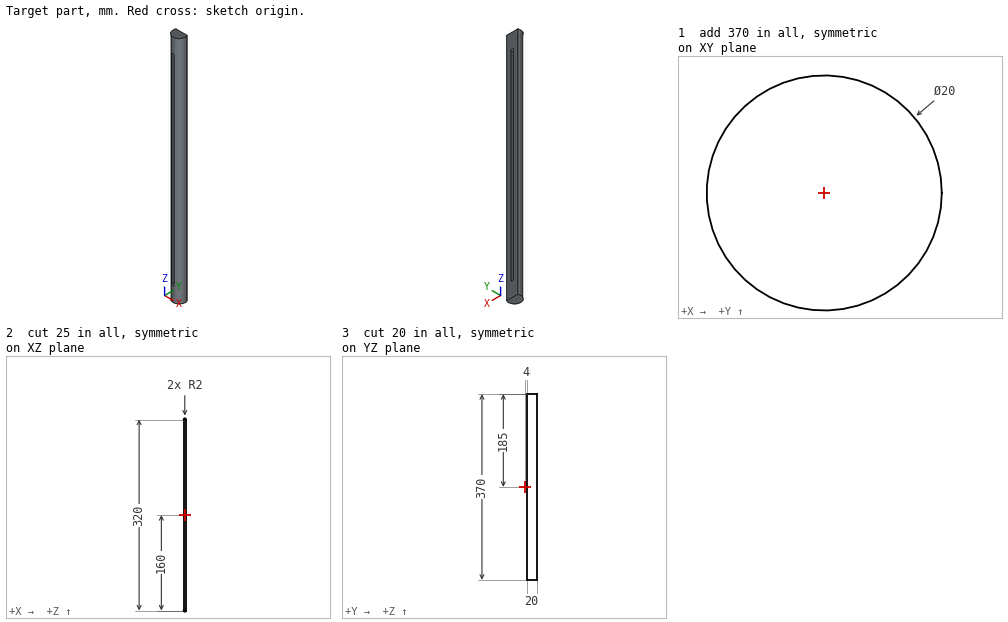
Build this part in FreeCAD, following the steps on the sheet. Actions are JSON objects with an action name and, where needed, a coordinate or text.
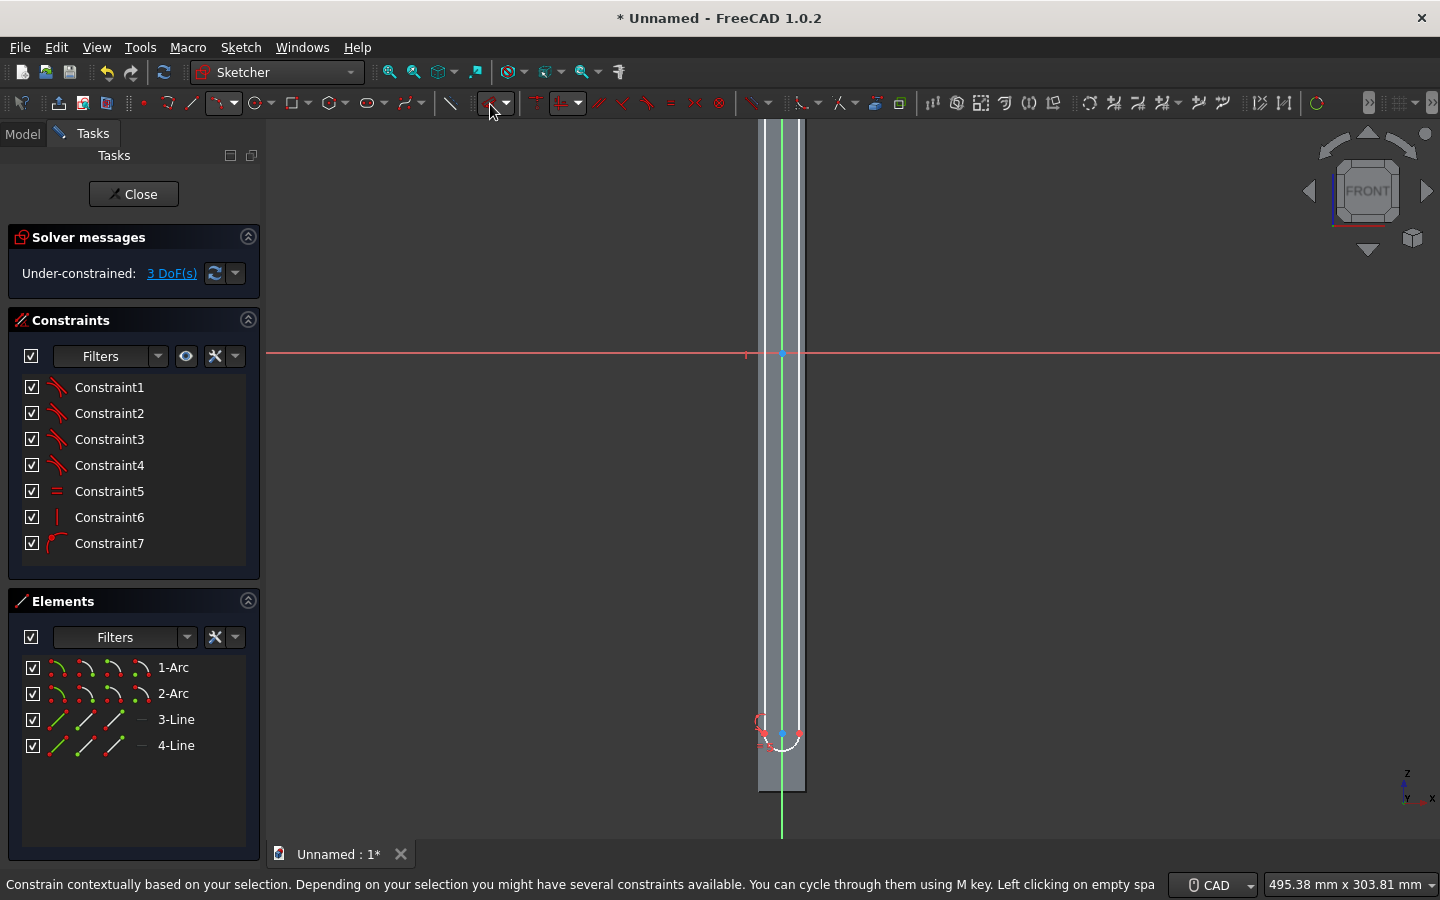
{"action": "scroll", "coordinate": [772, 748], "scroll_direction": "up", "scroll_amount": 11}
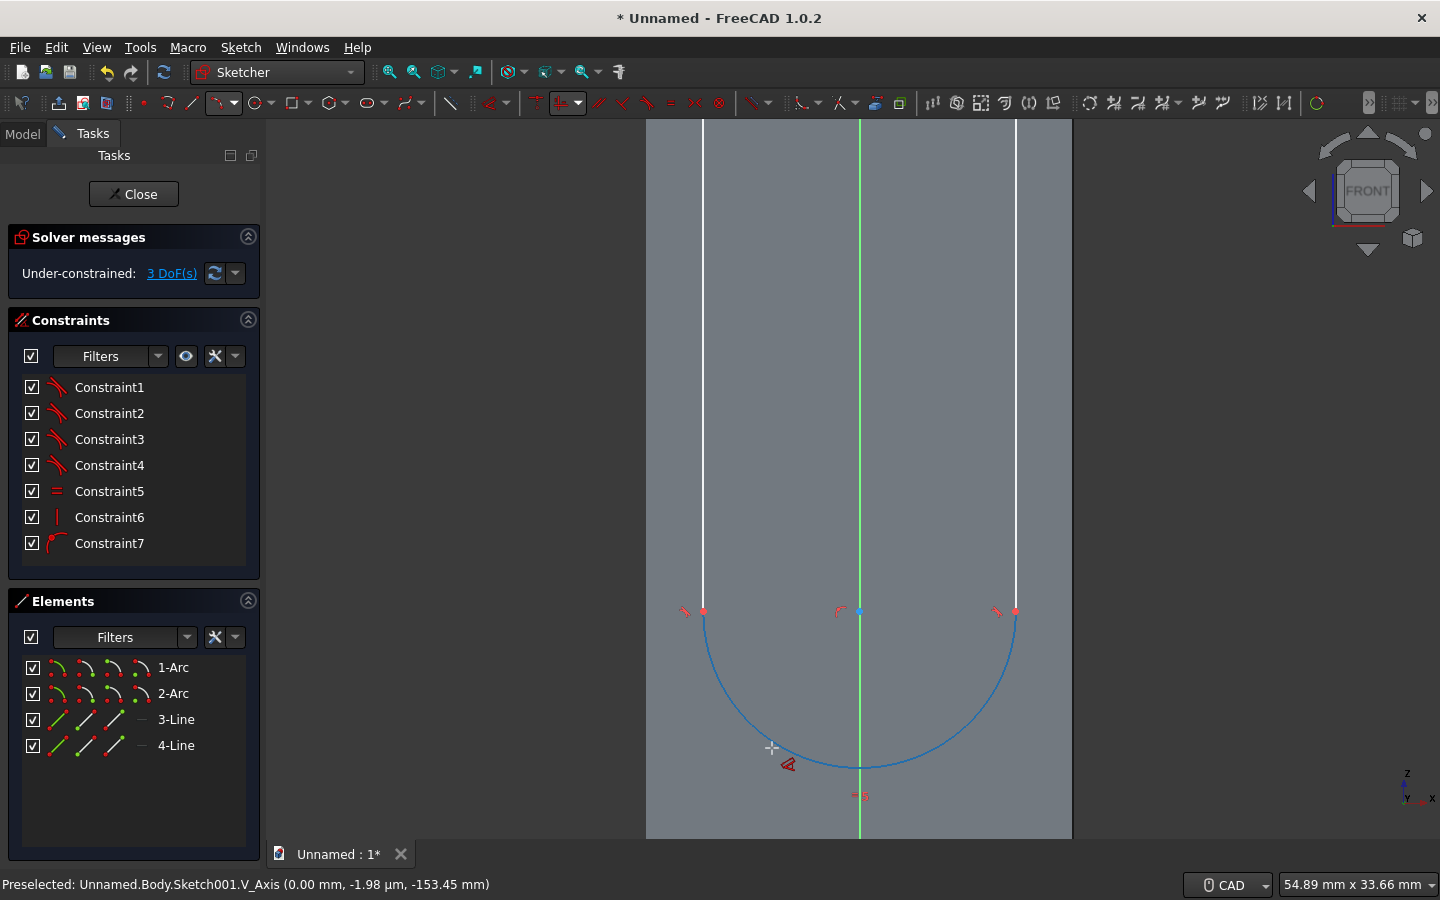
{"action": "left_click", "coordinate": [768, 738]}
{"action": "left_click", "coordinate": [749, 764]}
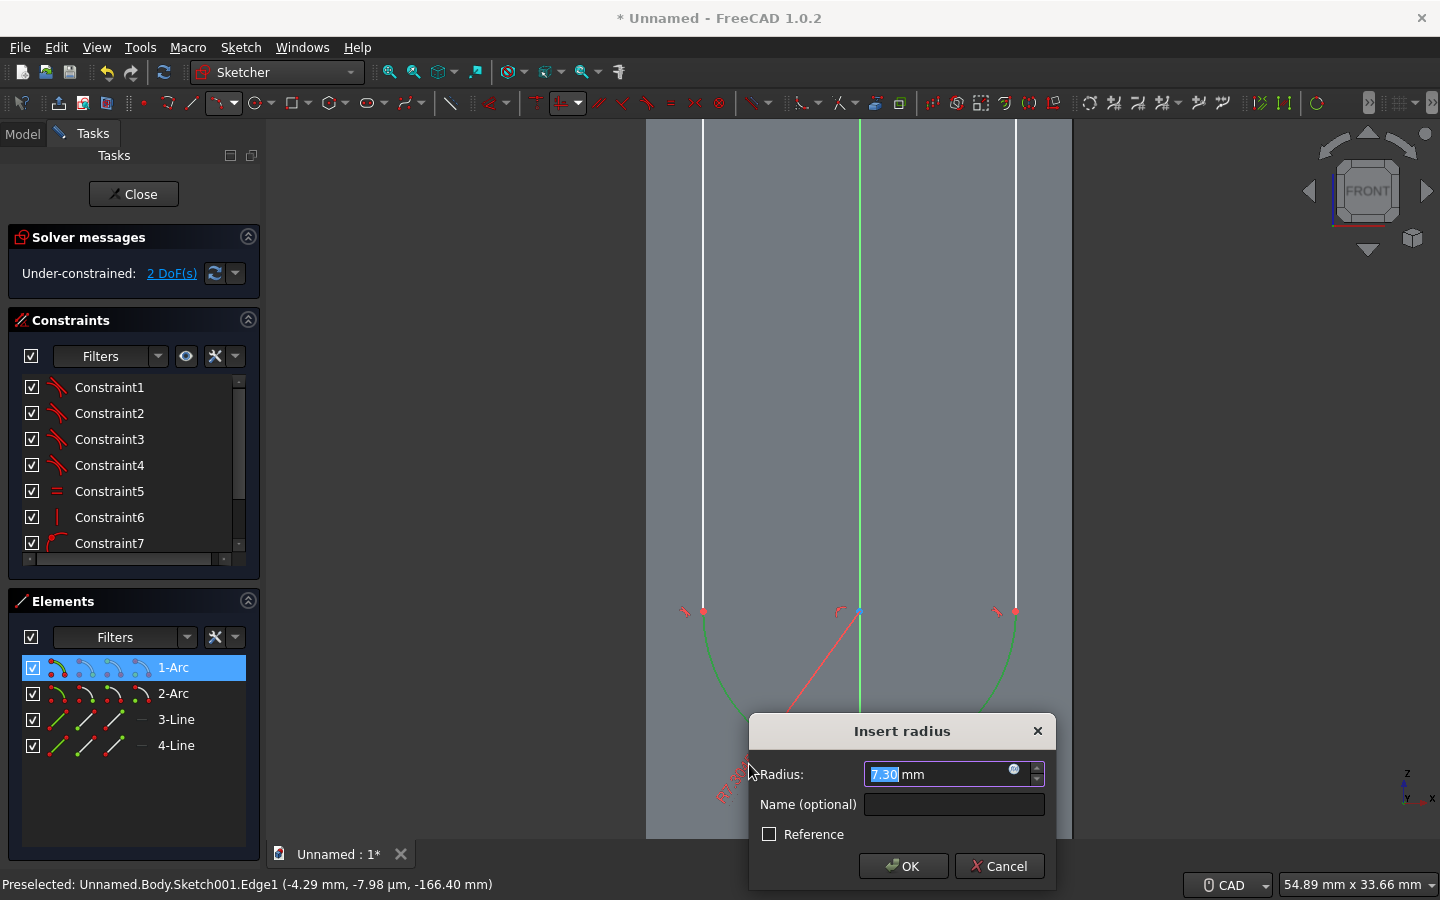
{"action": "type", "text": "2"}
{"action": "key", "text": "Return"}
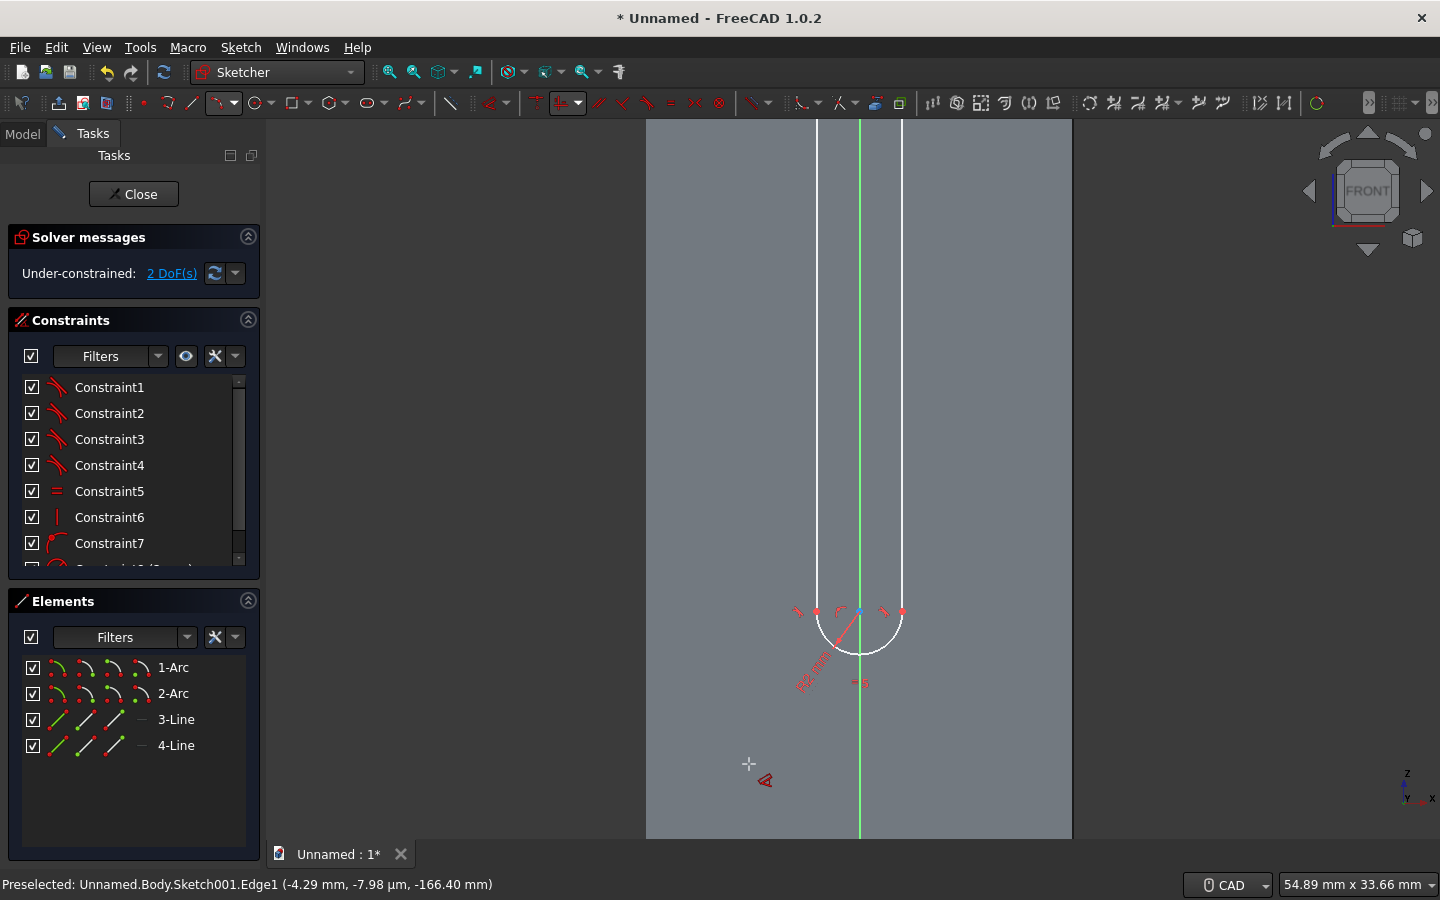
{"action": "scroll", "coordinate": [778, 744], "scroll_direction": "down", "scroll_amount": 13}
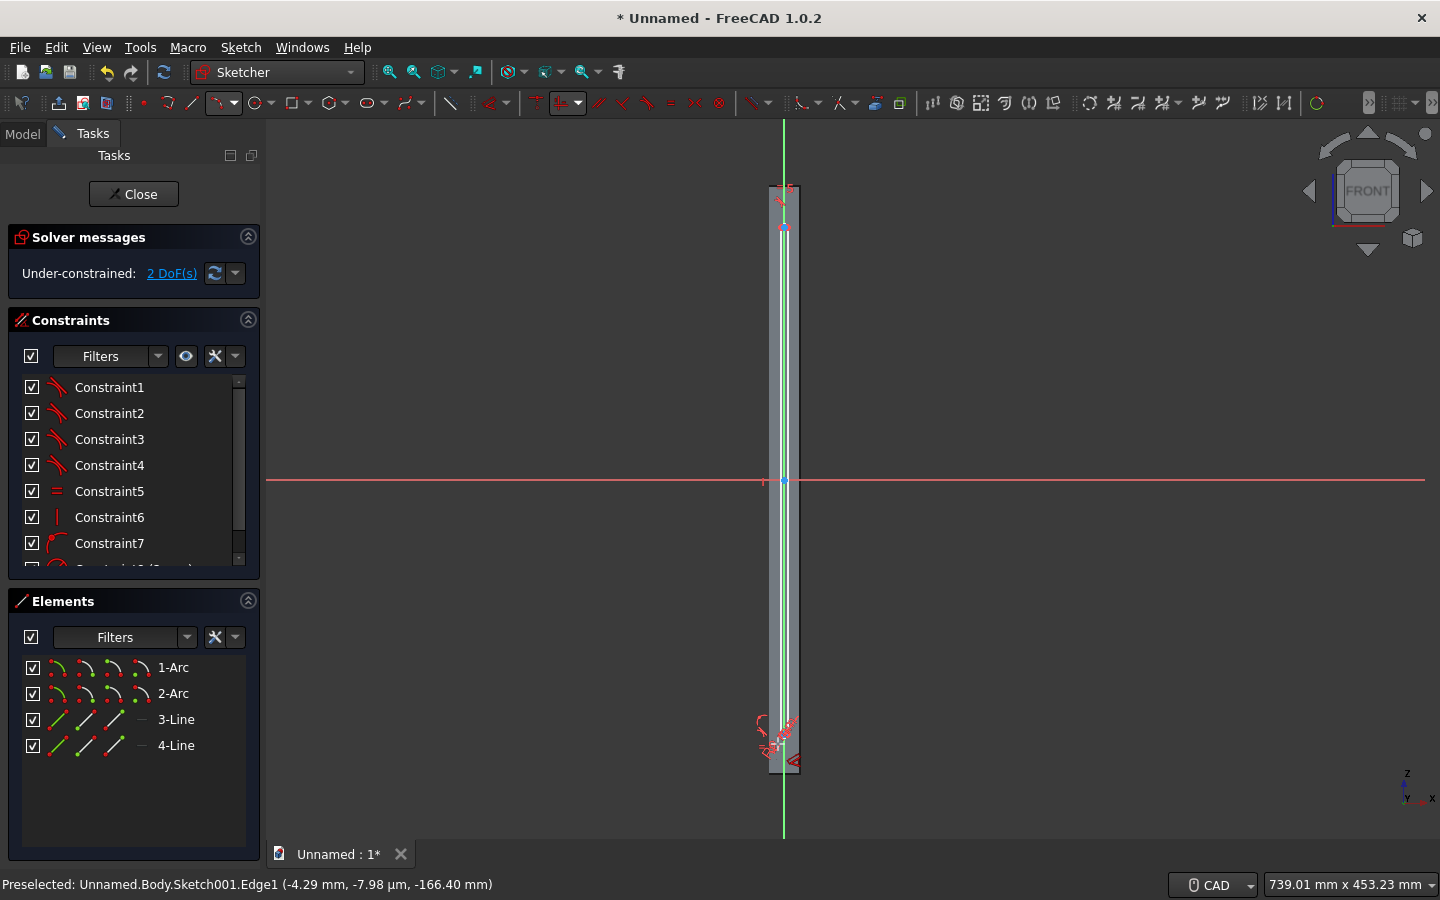
{"action": "scroll", "coordinate": [781, 583], "scroll_direction": "up", "scroll_amount": 8}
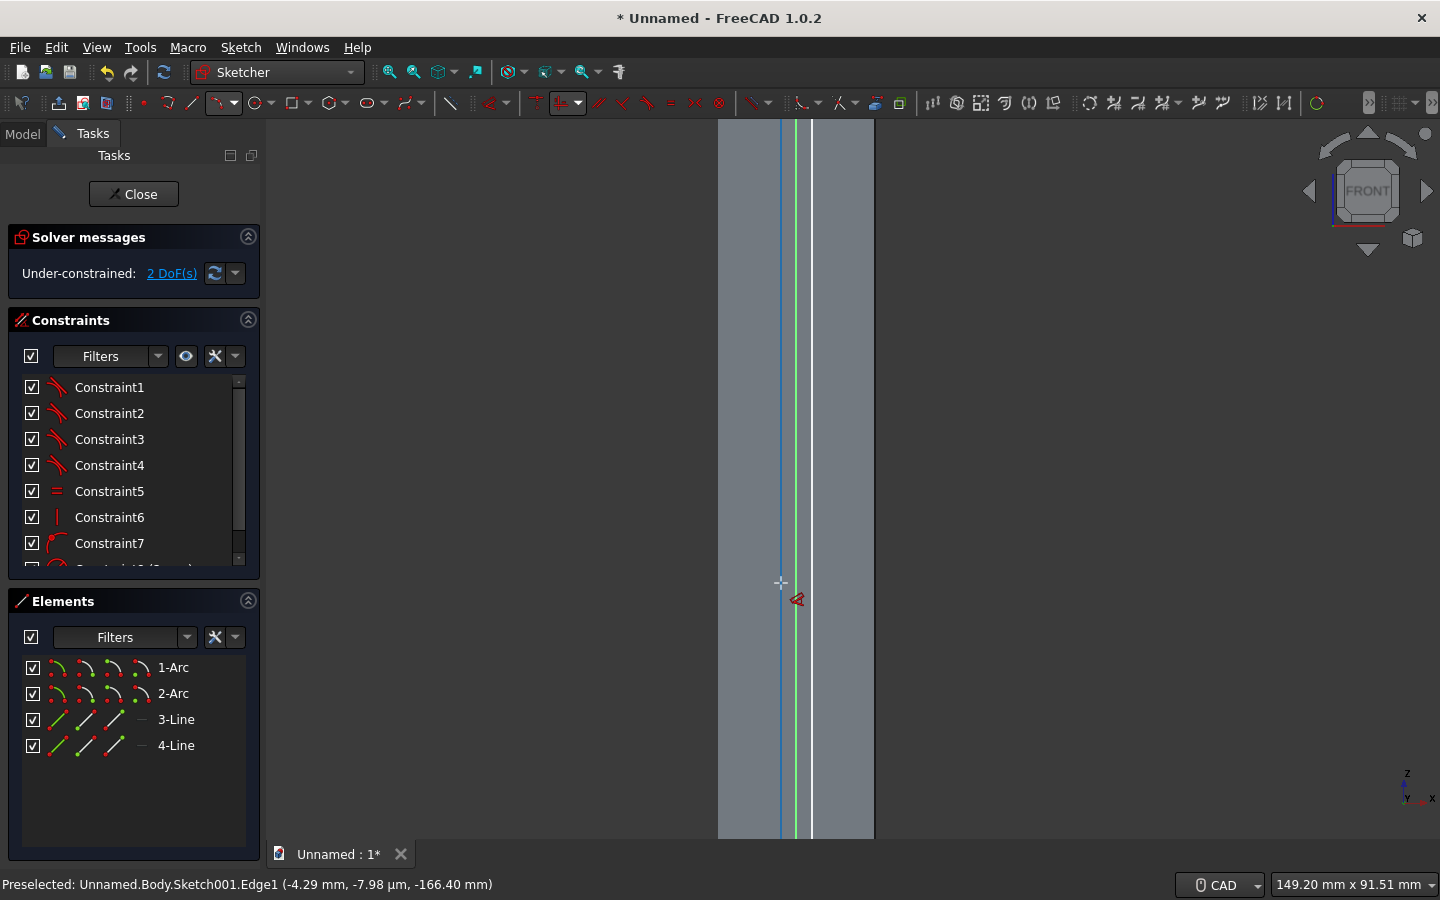
{"action": "left_click", "coordinate": [781, 579]}
{"action": "left_click", "coordinate": [747, 479]}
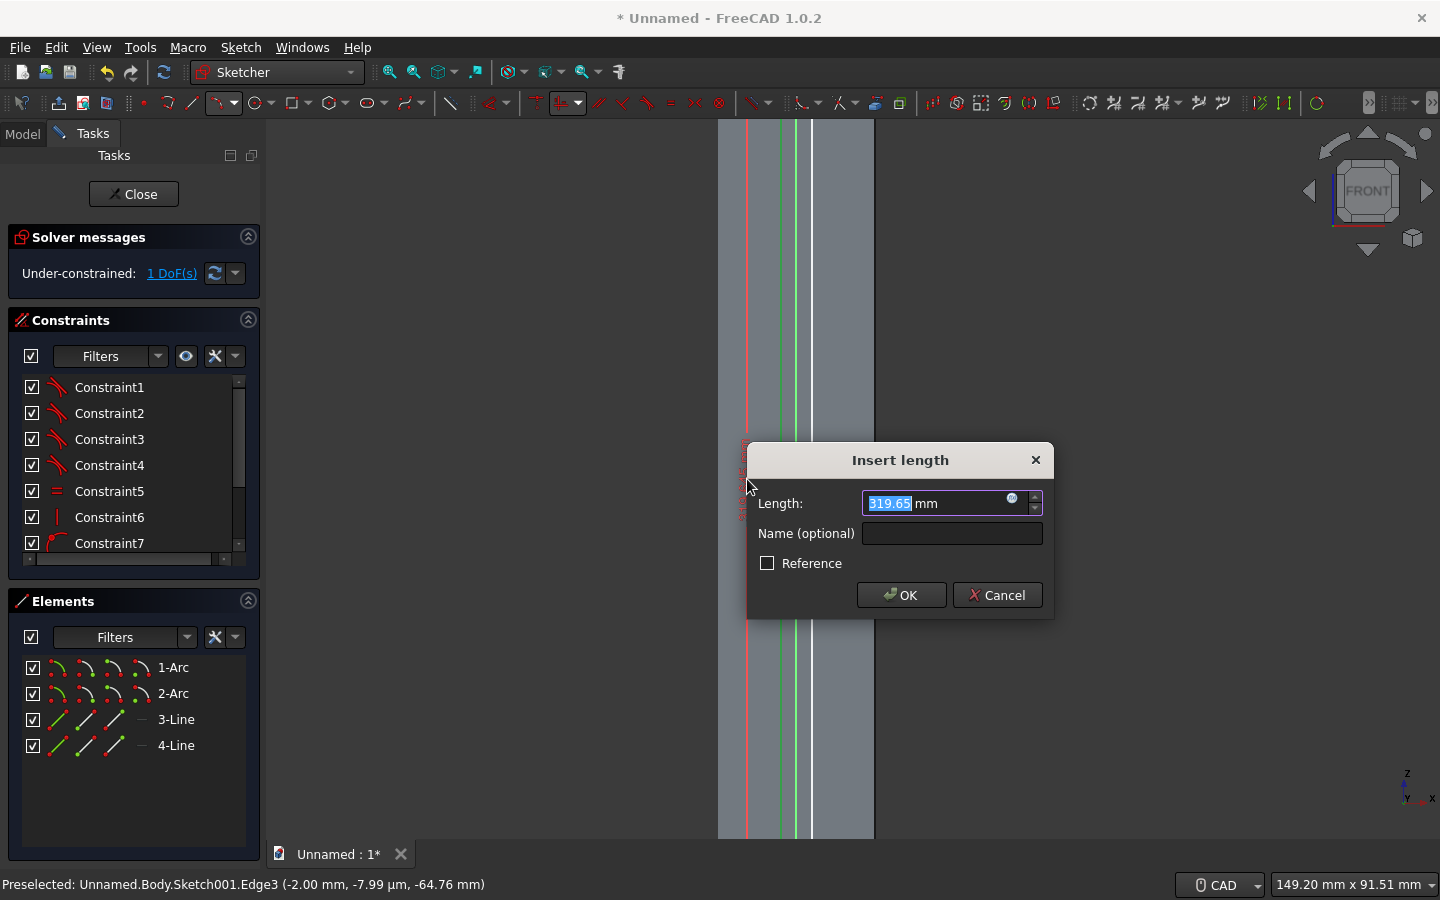
{"action": "type", "text": "320"}
{"action": "key", "text": "Return"}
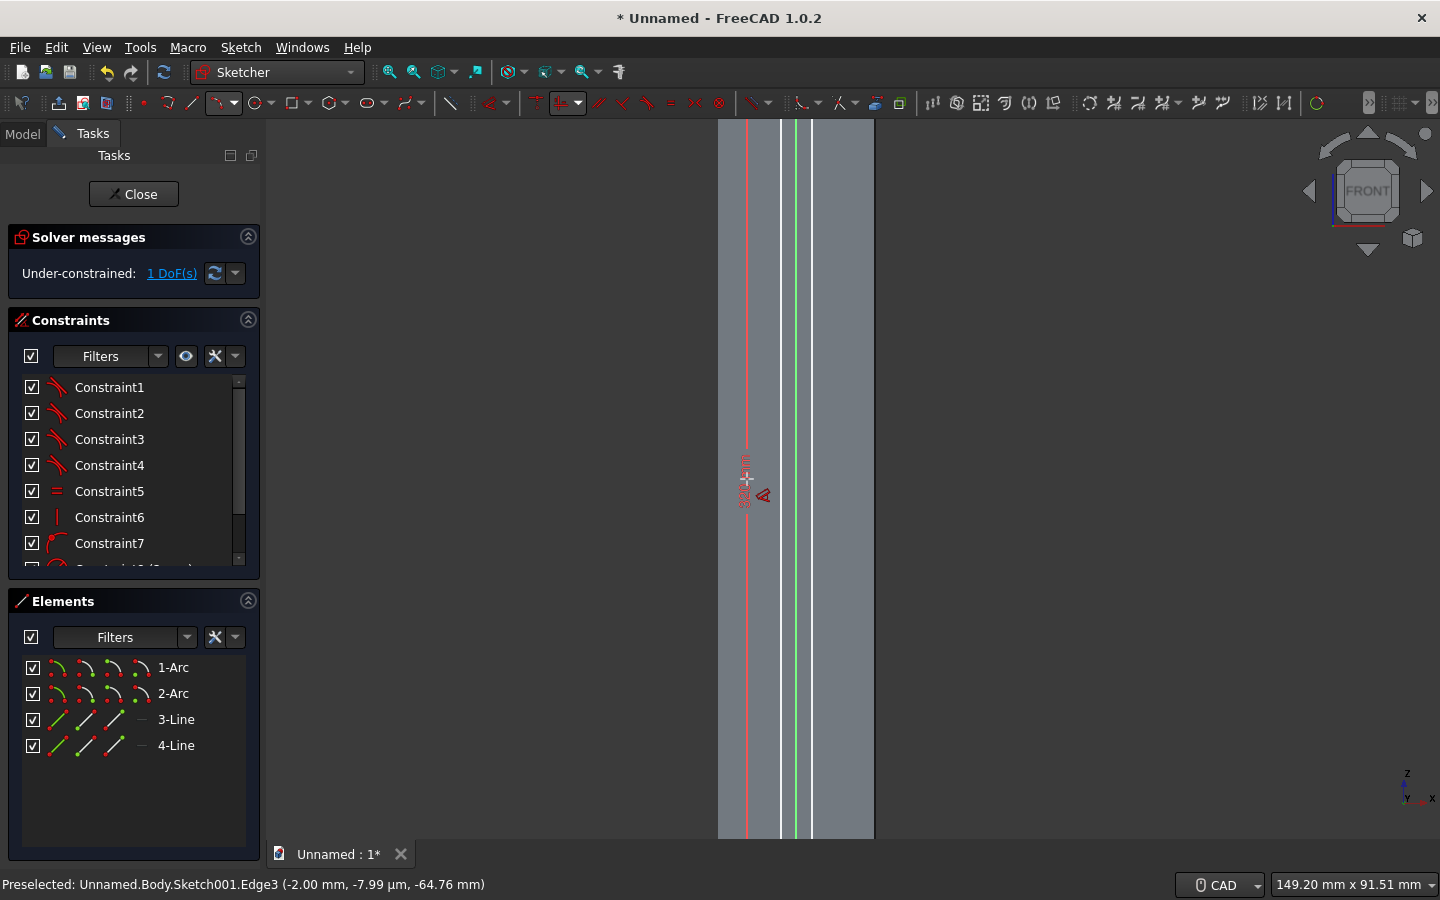
{"action": "scroll", "coordinate": [781, 582], "scroll_direction": "down", "scroll_amount": 8}